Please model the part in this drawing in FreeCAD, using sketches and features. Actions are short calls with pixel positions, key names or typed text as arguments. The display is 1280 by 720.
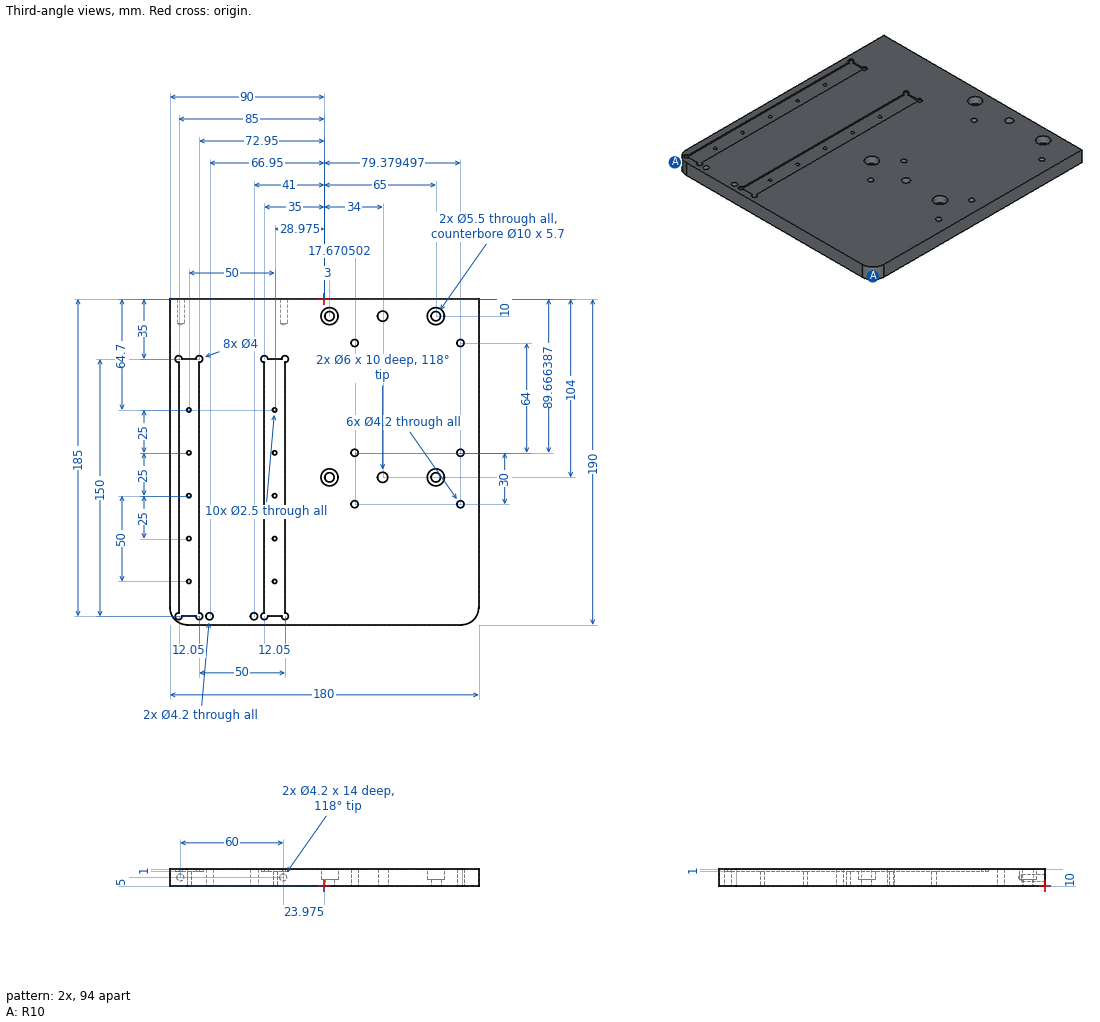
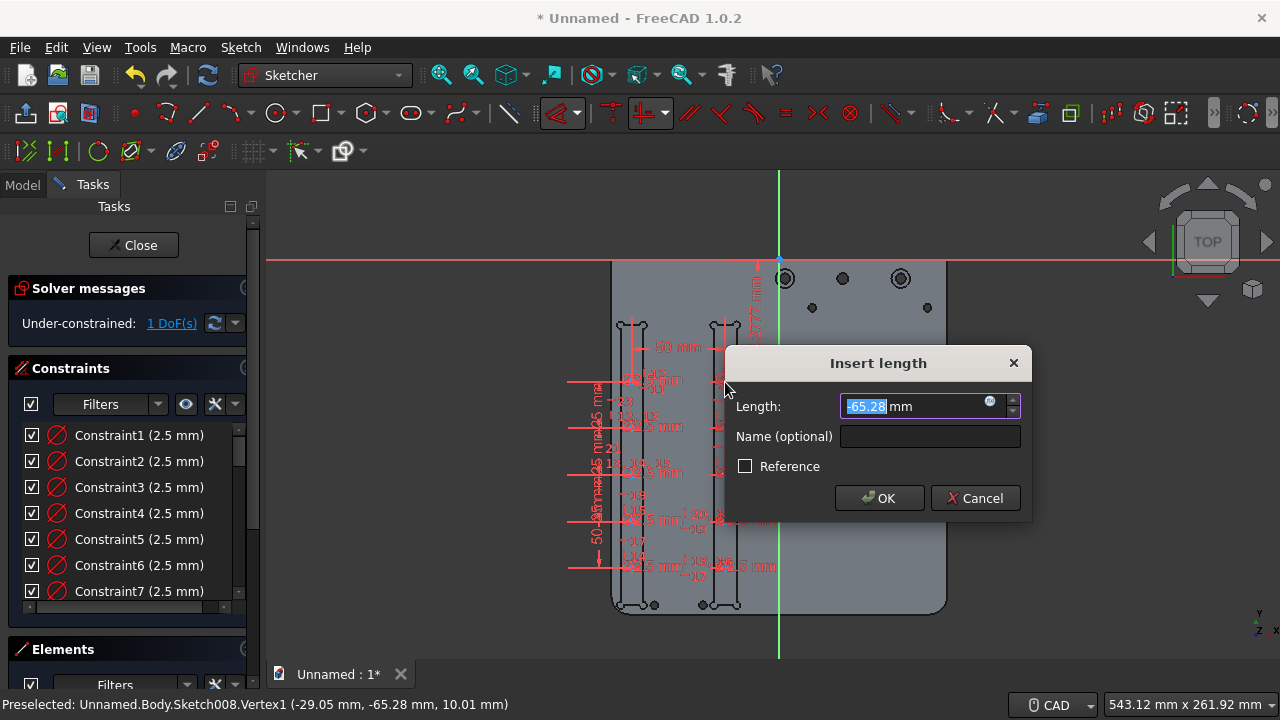
text(-64.7)
key(Return)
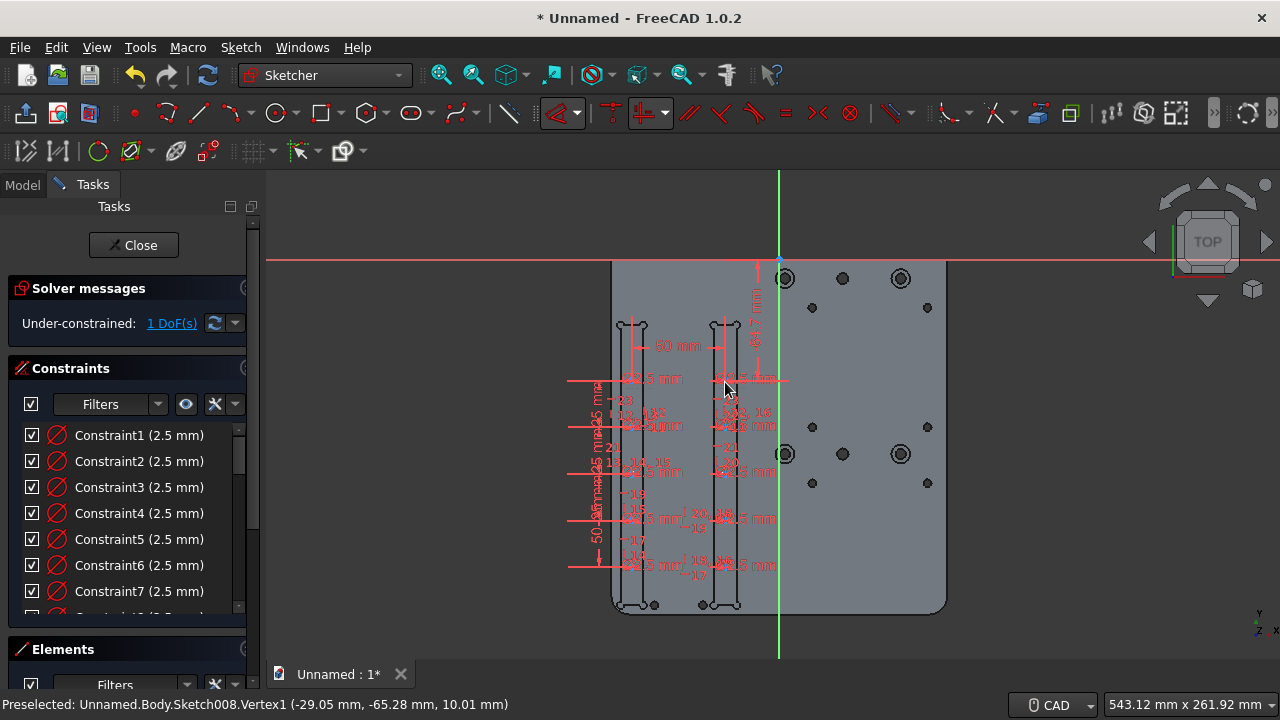
click(725, 381)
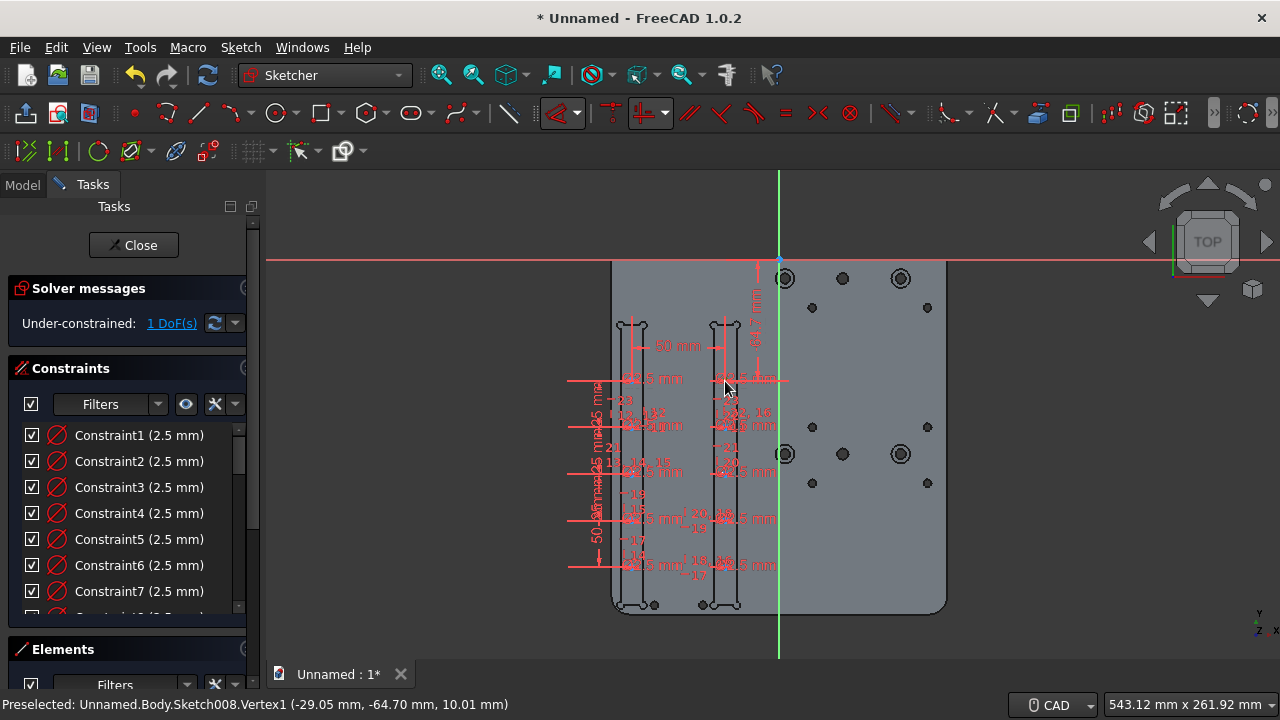
key(l)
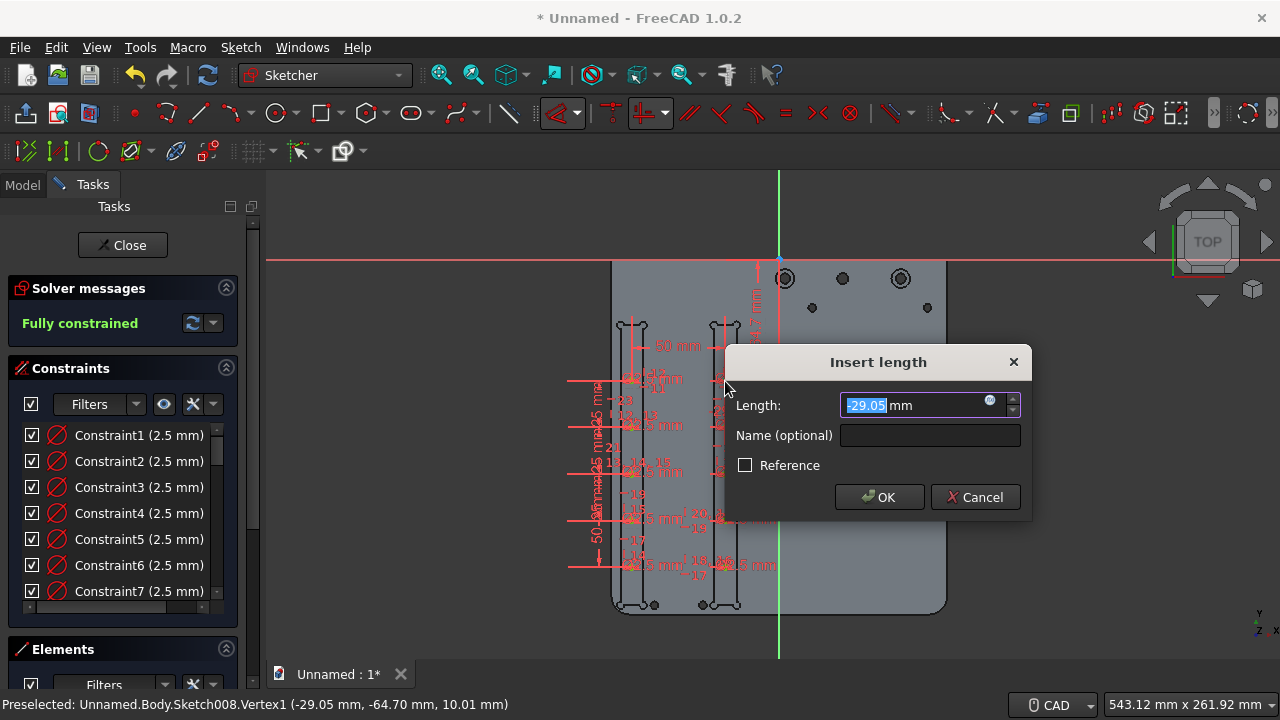
text(-28.975)
key(Return)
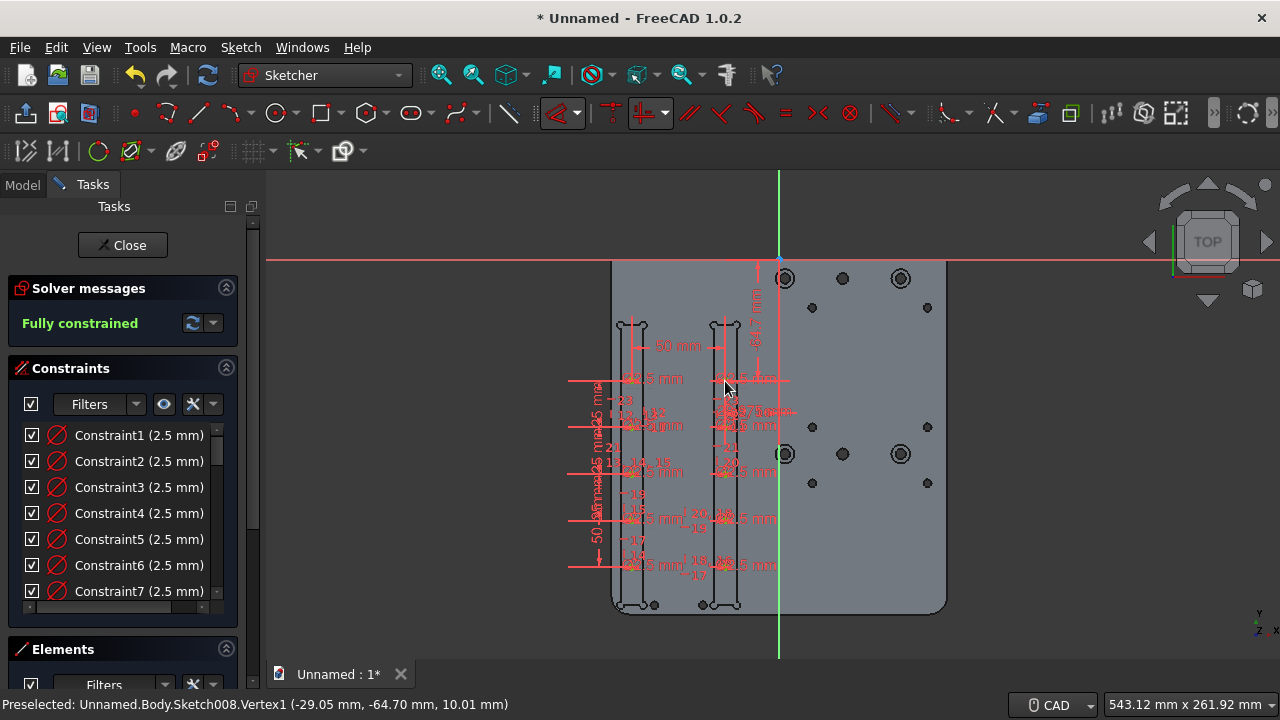
click(123, 245)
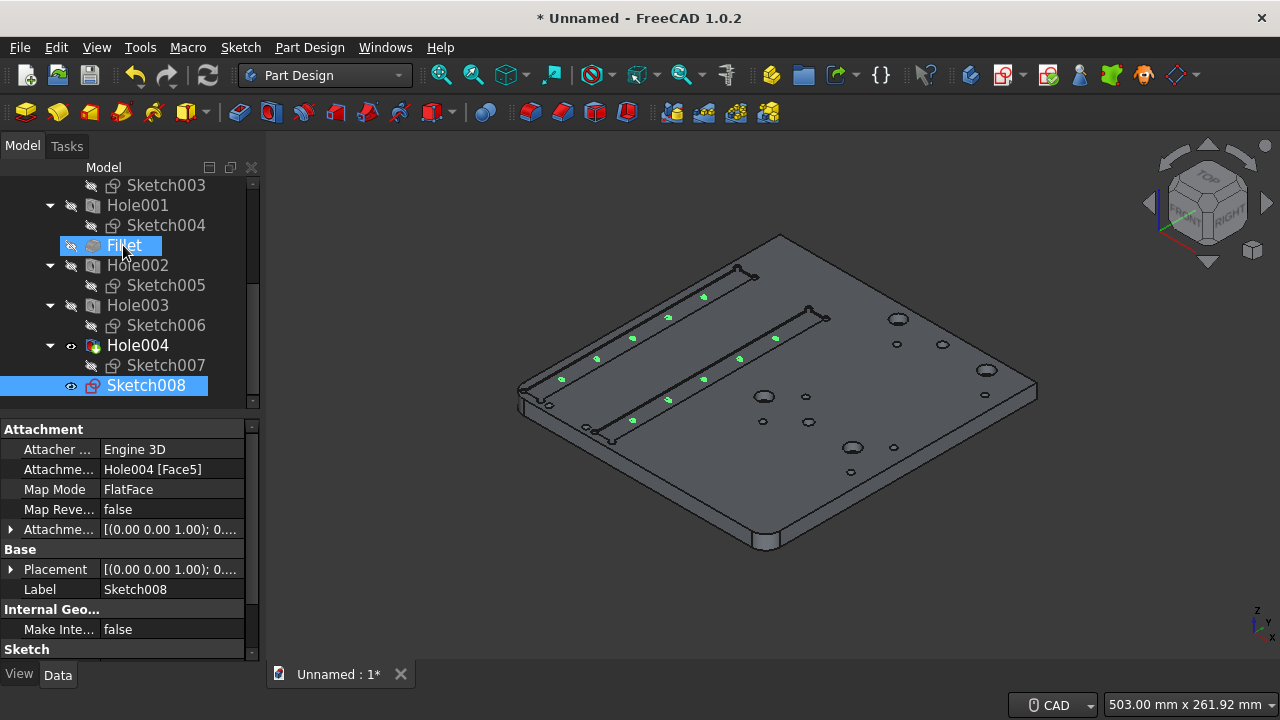
click(272, 112)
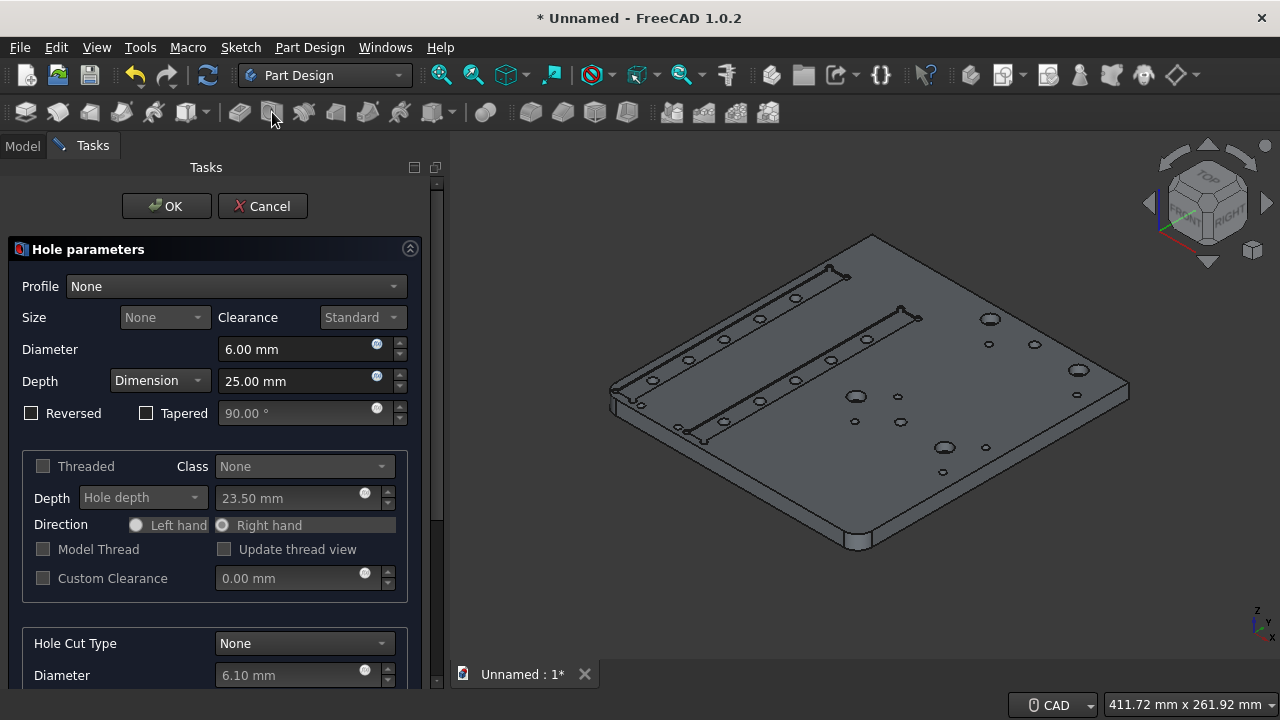
triple_click(305, 349)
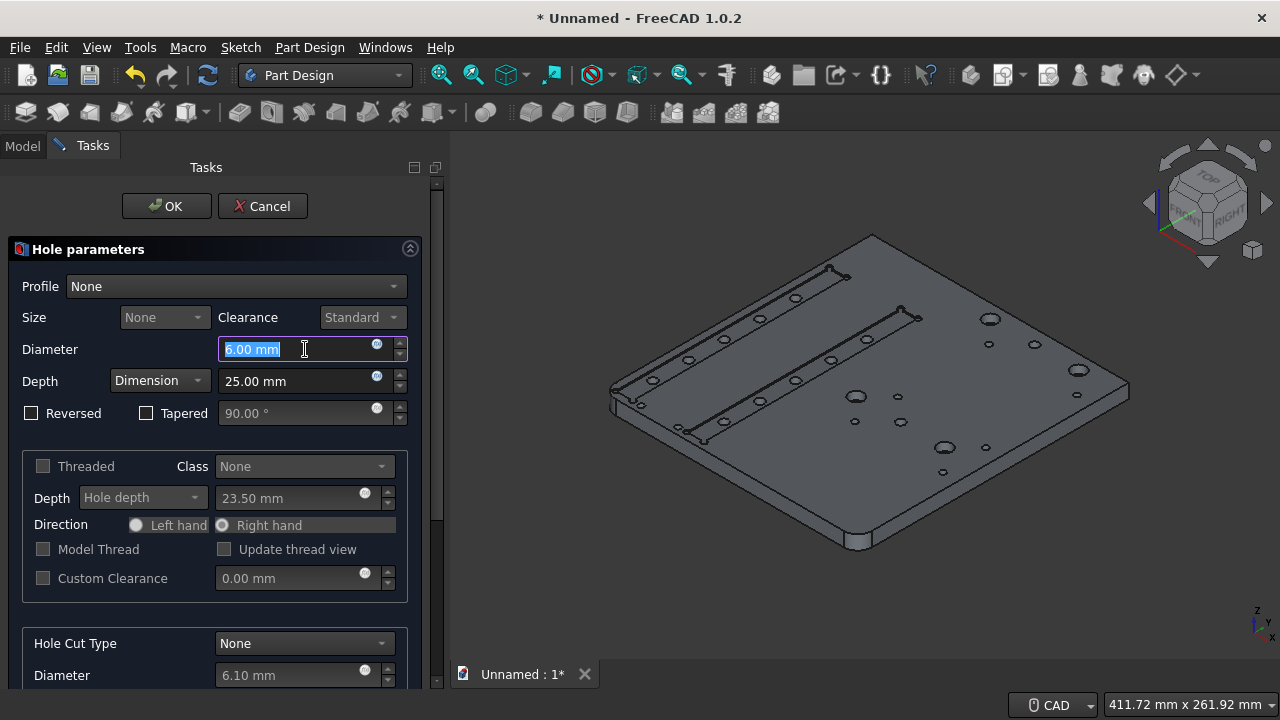
text(2.5)
key(Tab)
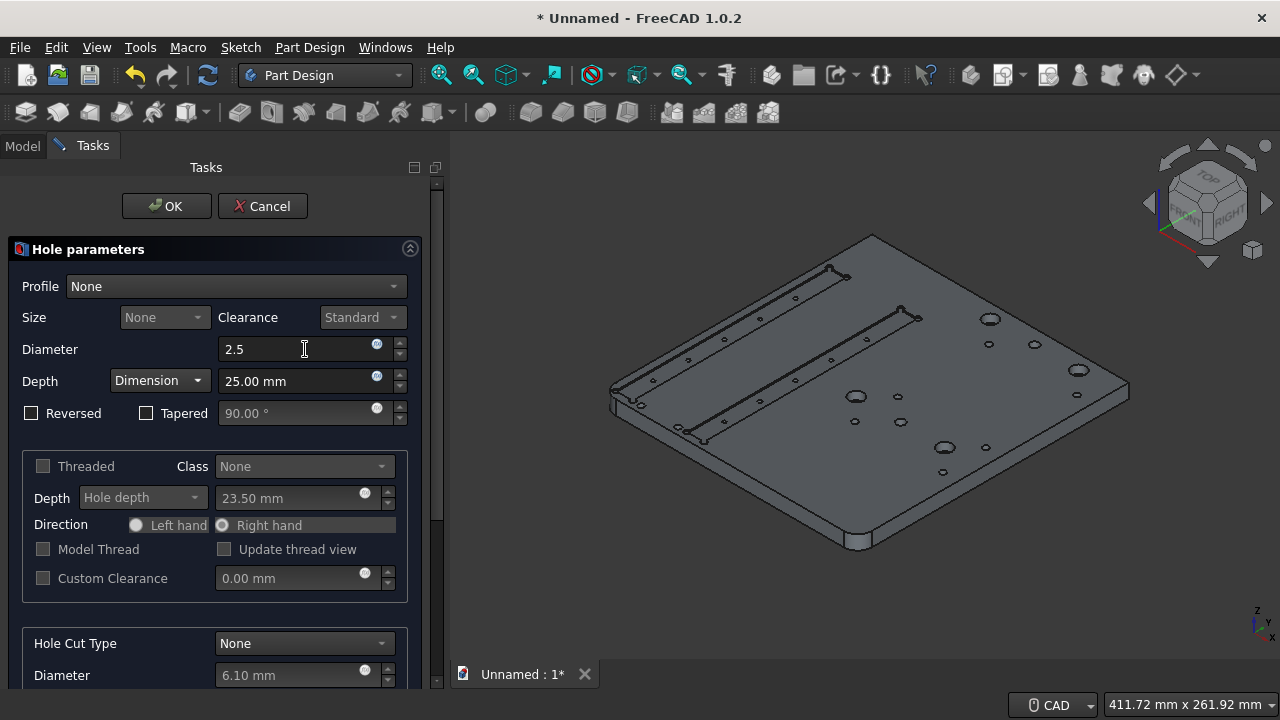
click(161, 380)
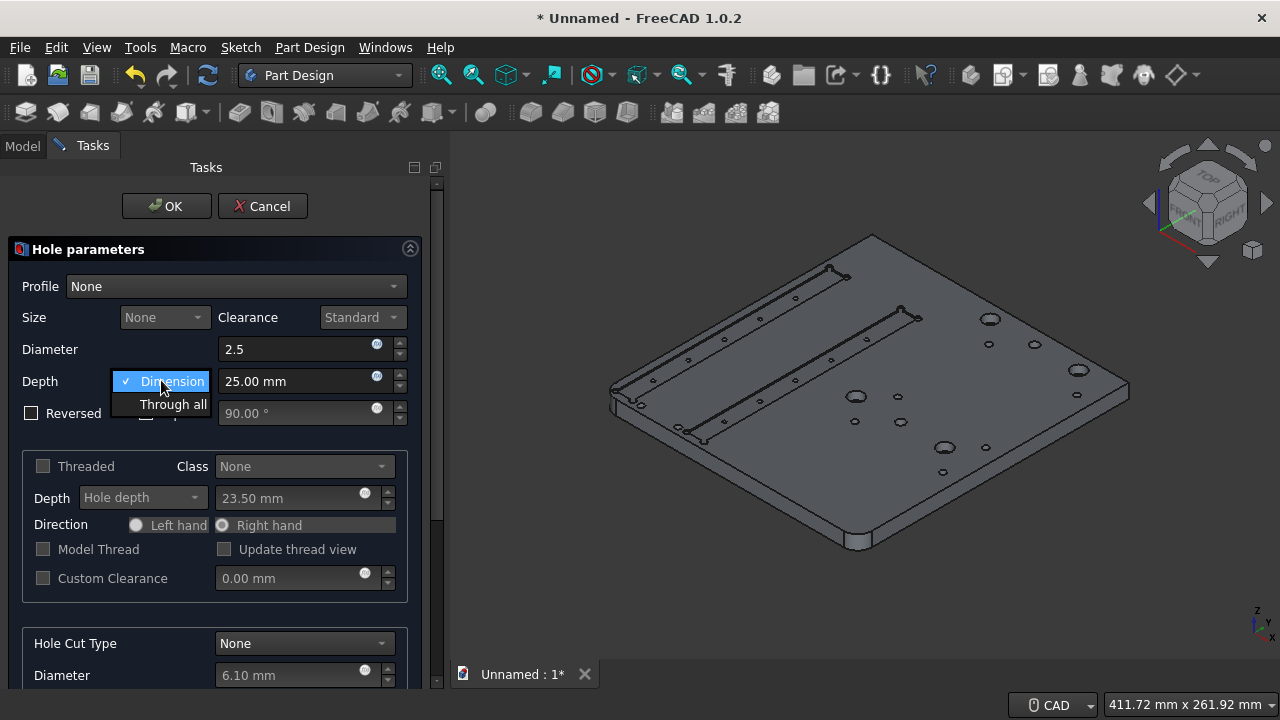
click(160, 404)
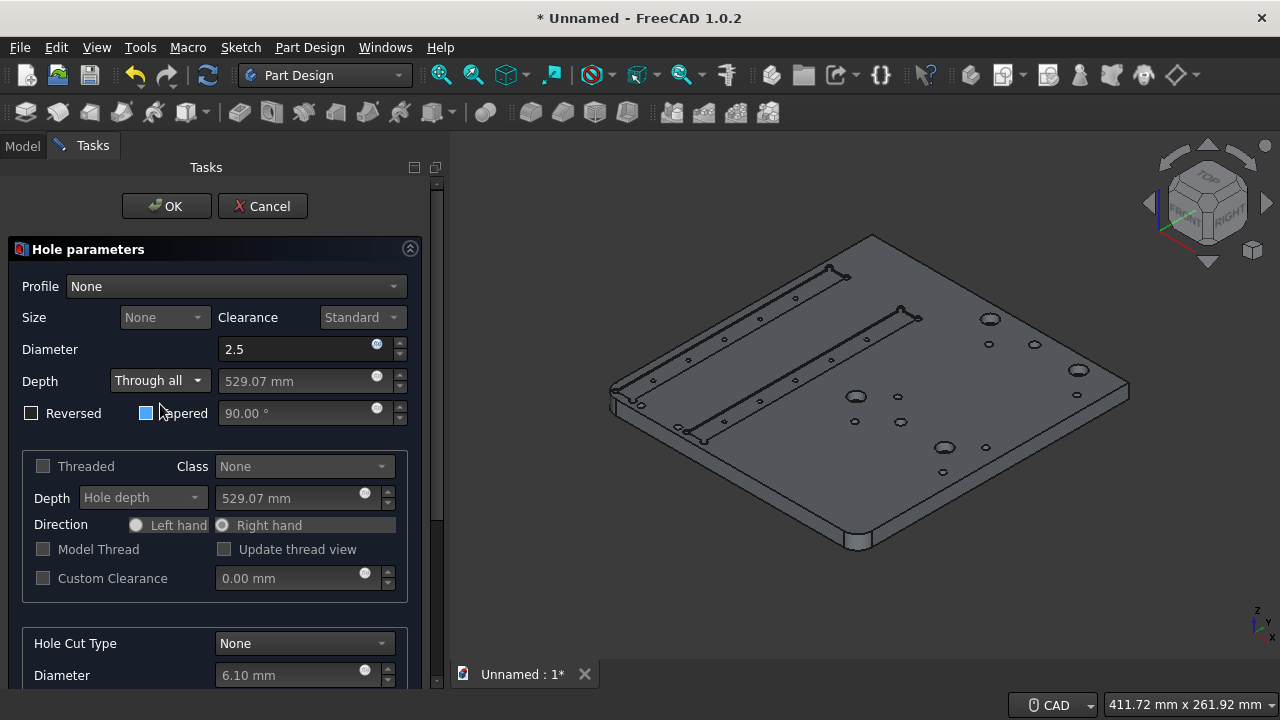
click(167, 206)